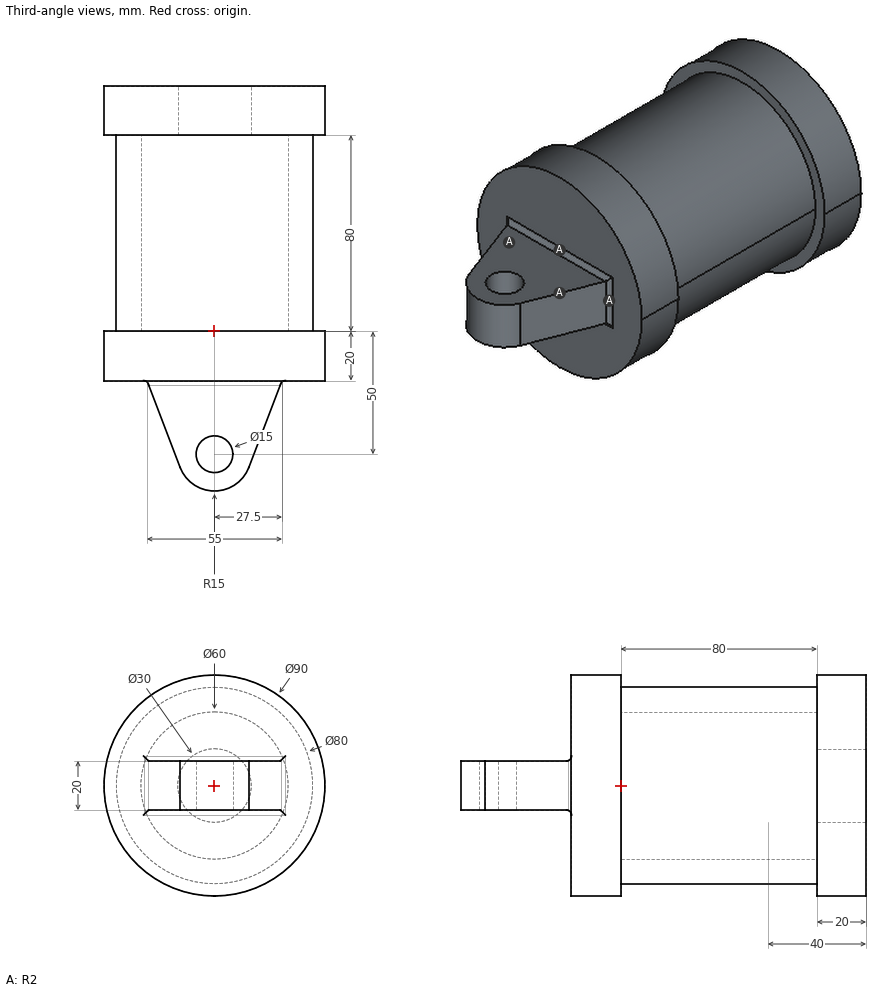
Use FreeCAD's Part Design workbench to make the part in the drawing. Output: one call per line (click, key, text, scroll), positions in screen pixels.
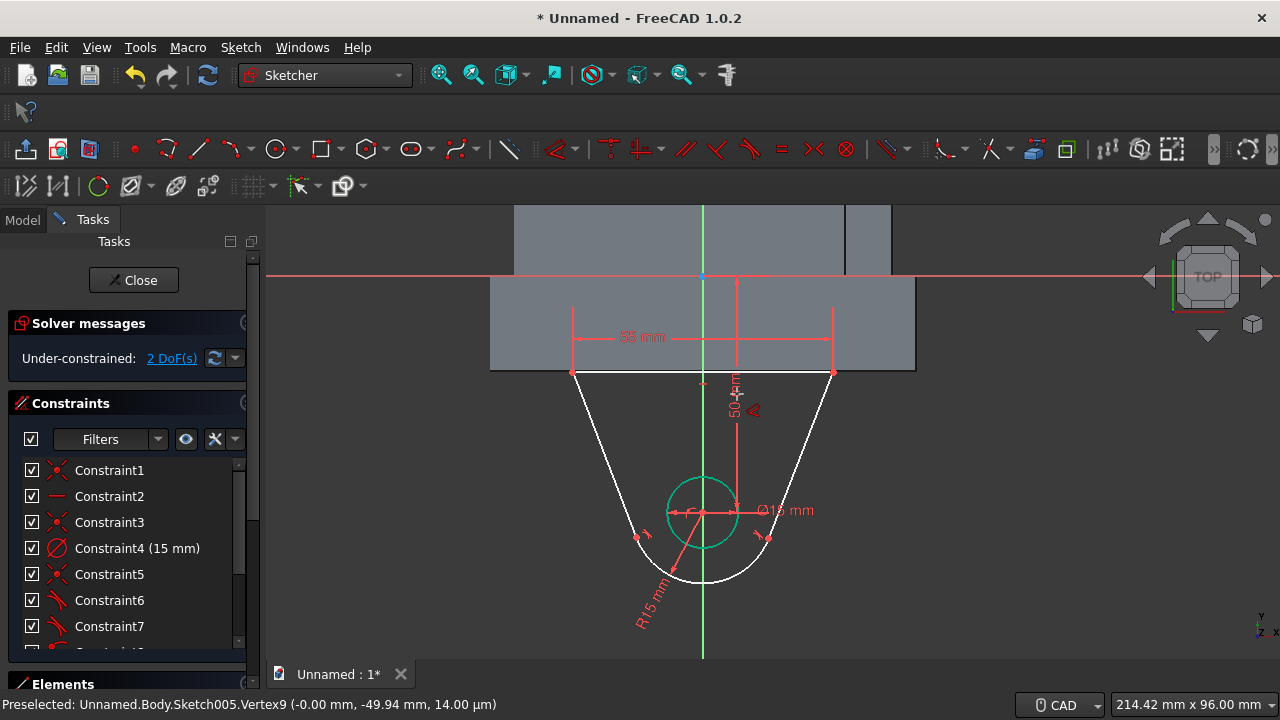
click(833, 372)
click(867, 324)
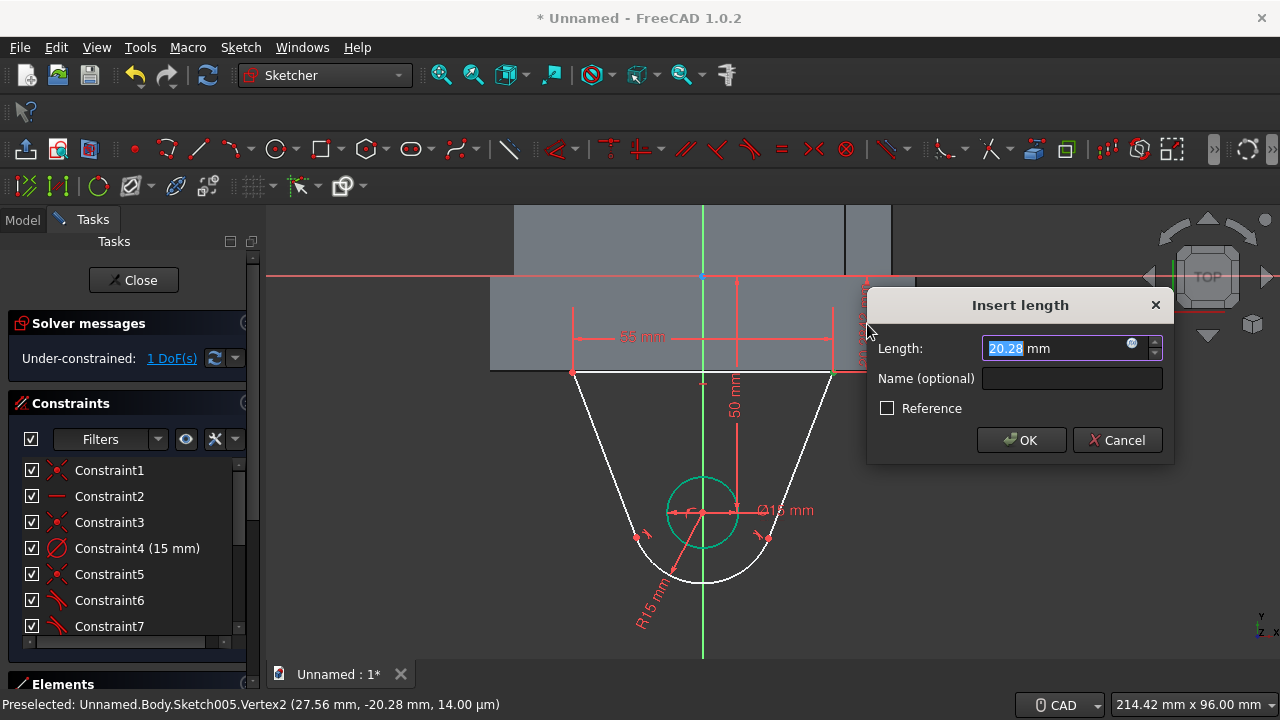
text(20)
key(Return)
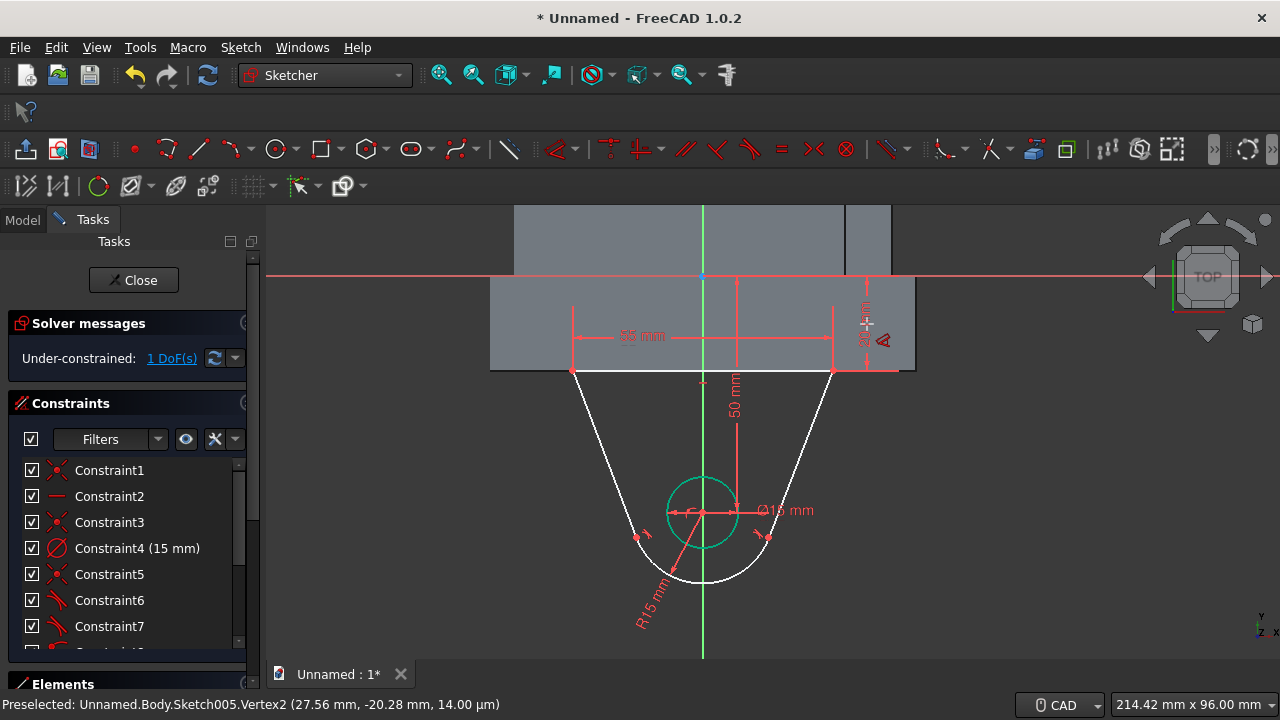
click(833, 371)
click(768, 242)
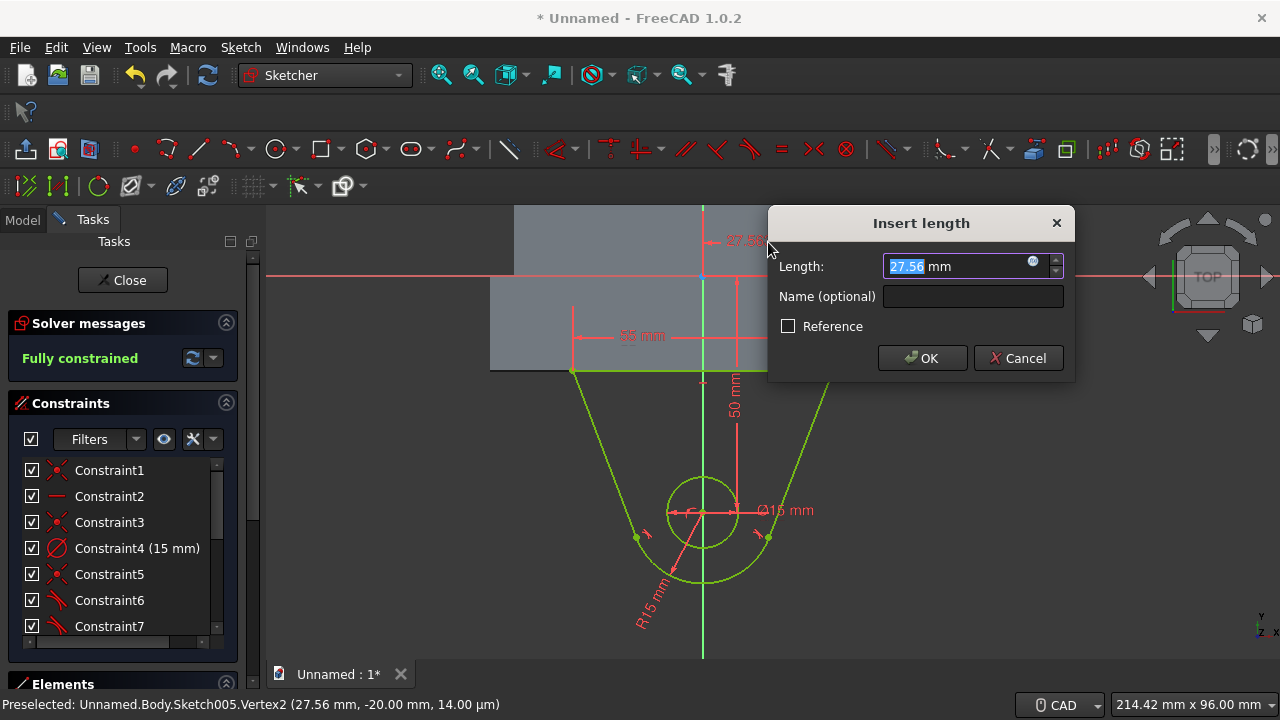
text(27.5)
key(Return)
key(Escape)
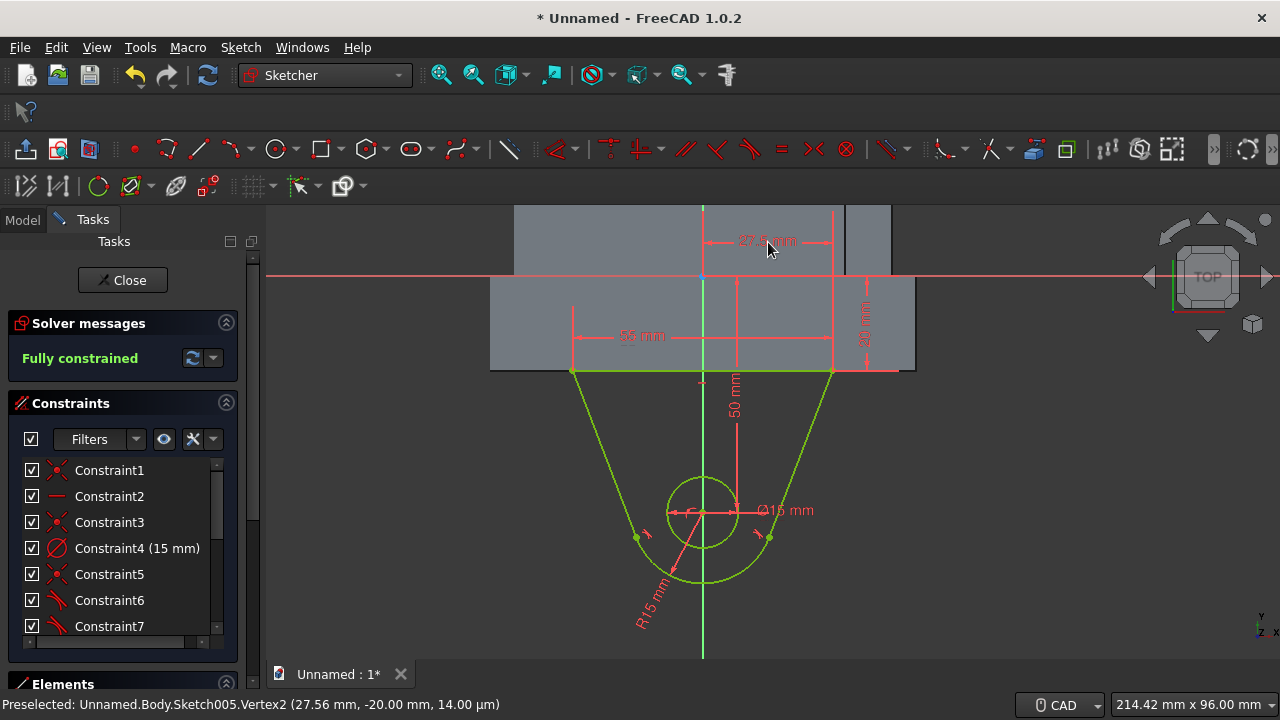
click(123, 280)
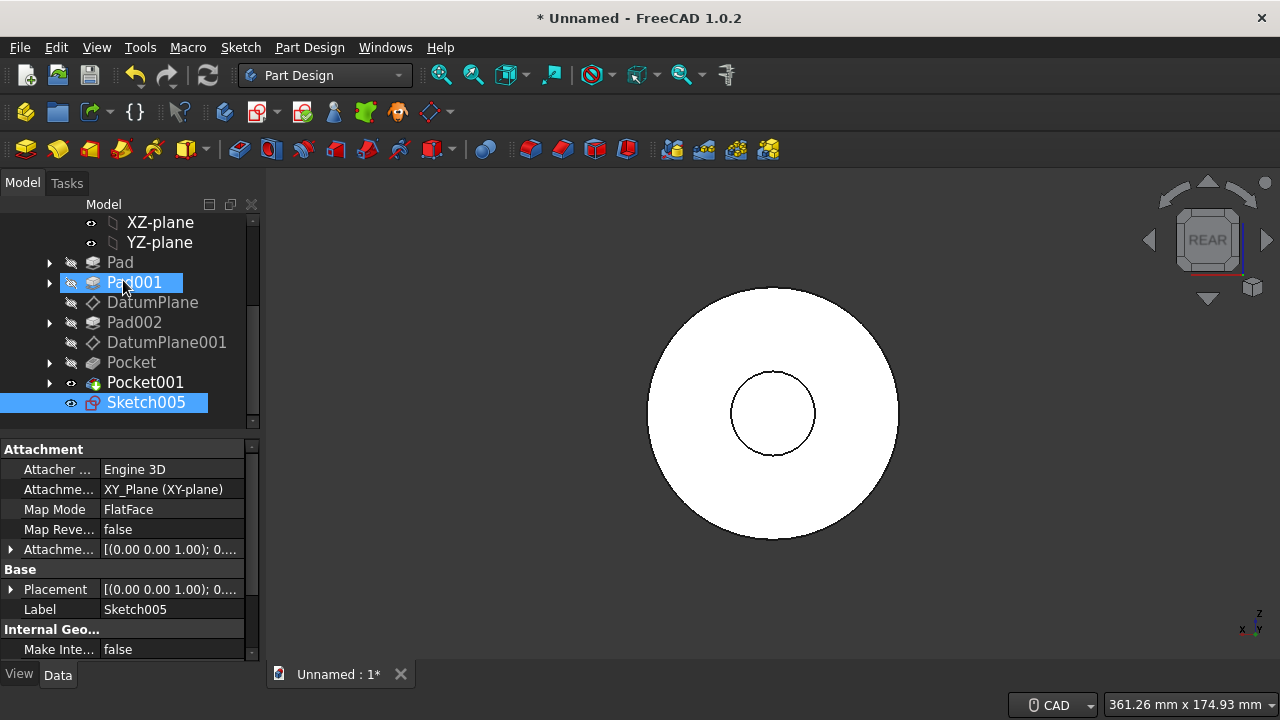
click(26, 150)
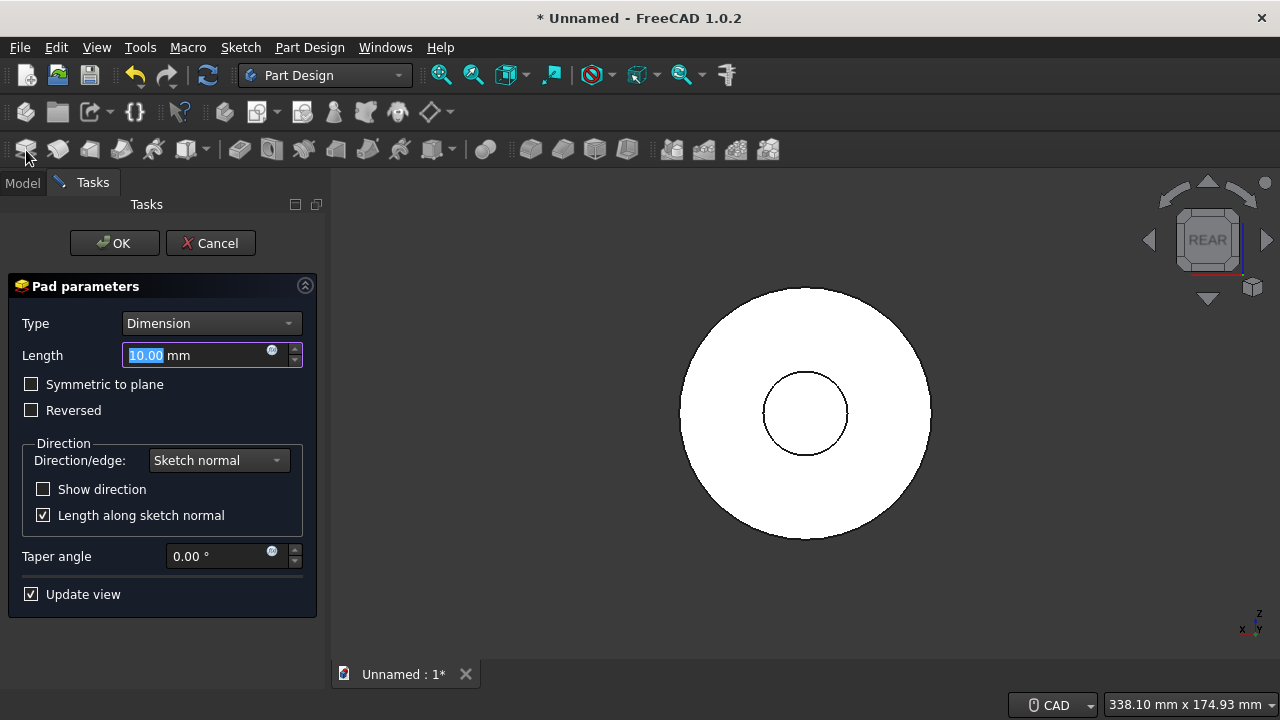
text(20)
key(Tab)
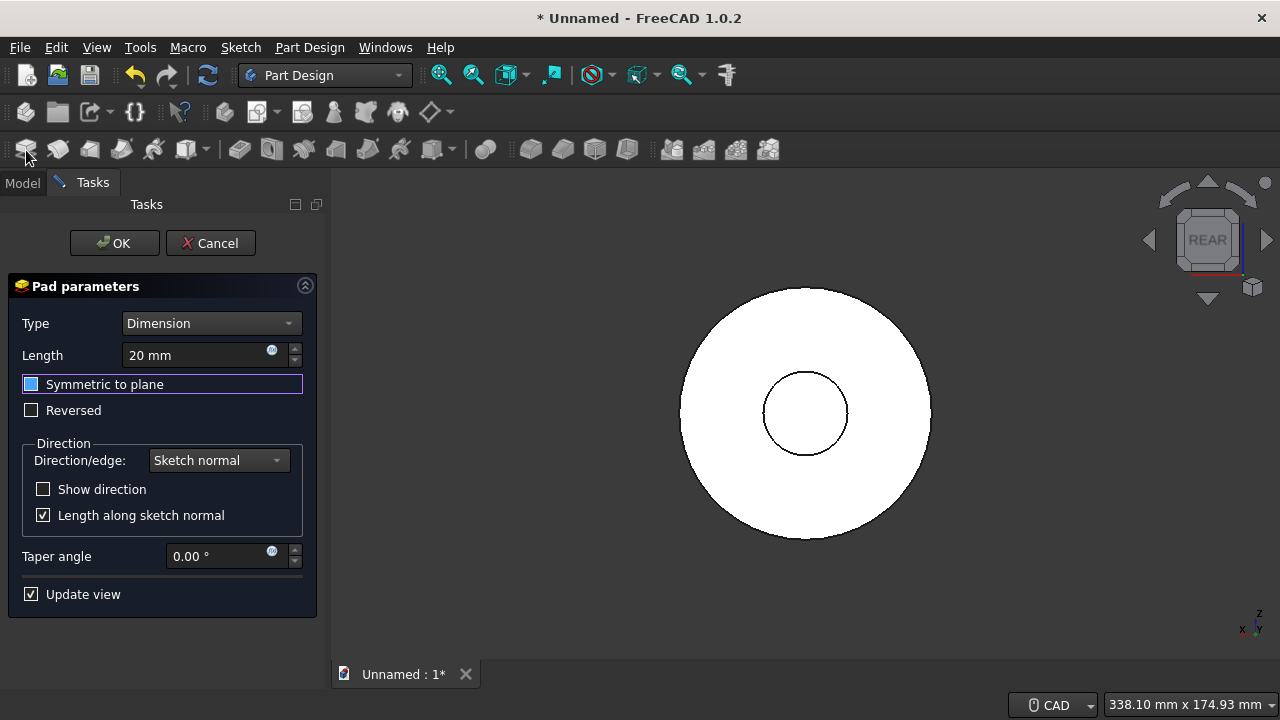
click(30, 384)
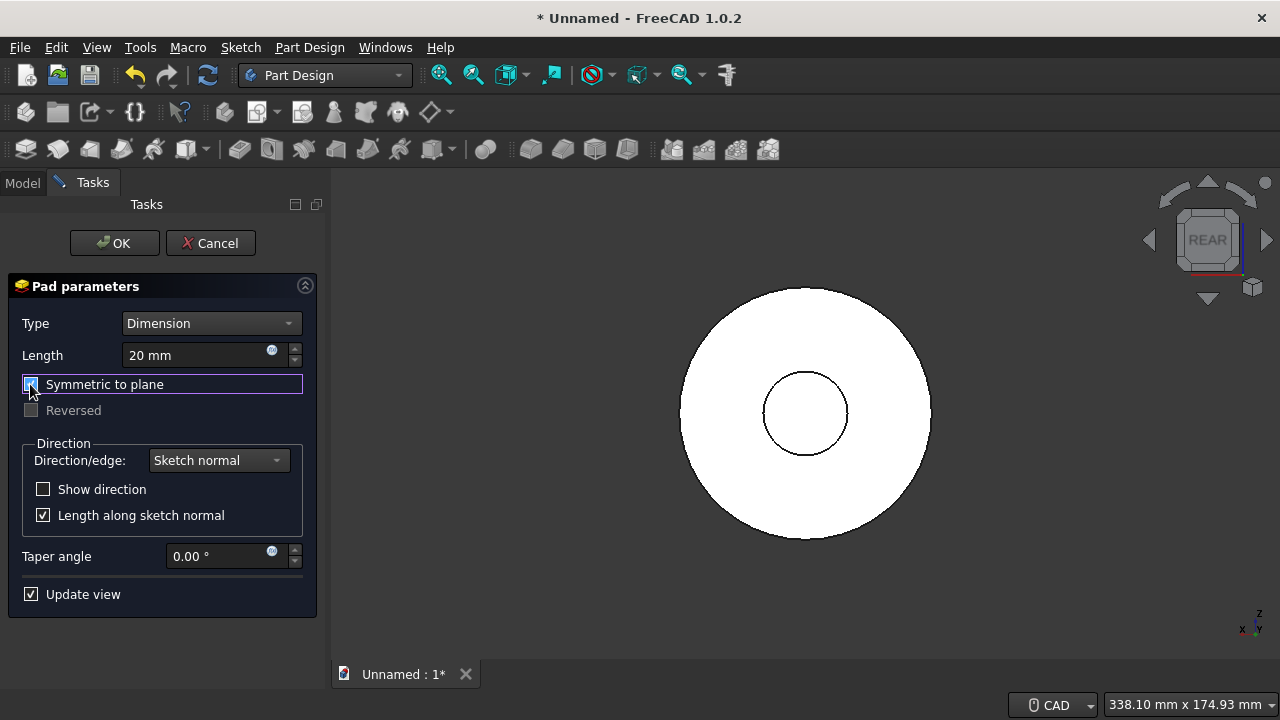
click(115, 243)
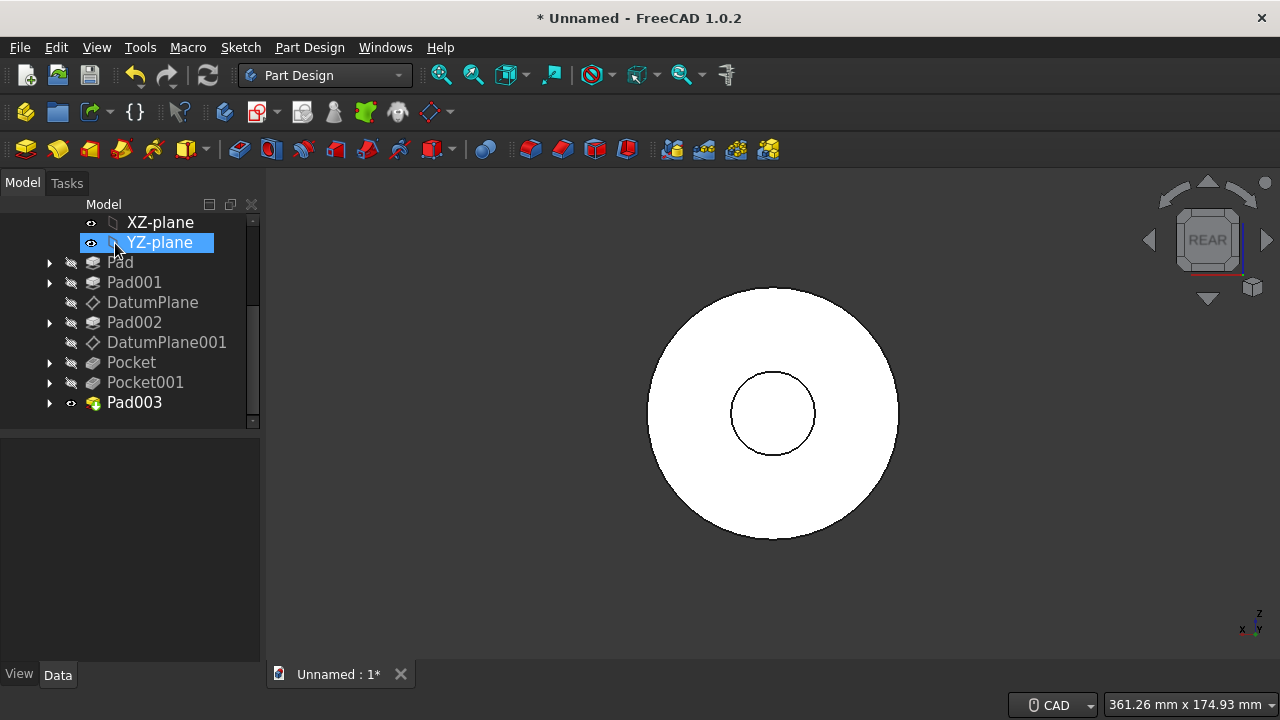
key(0)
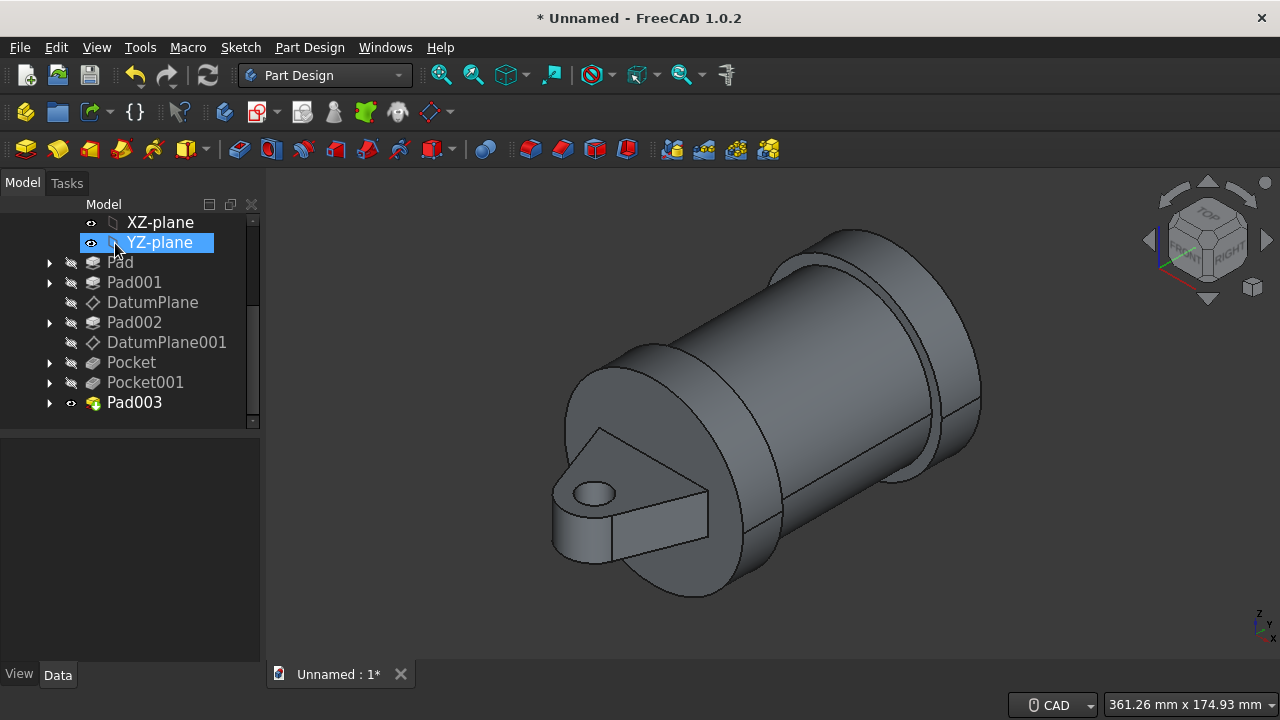
click(442, 76)